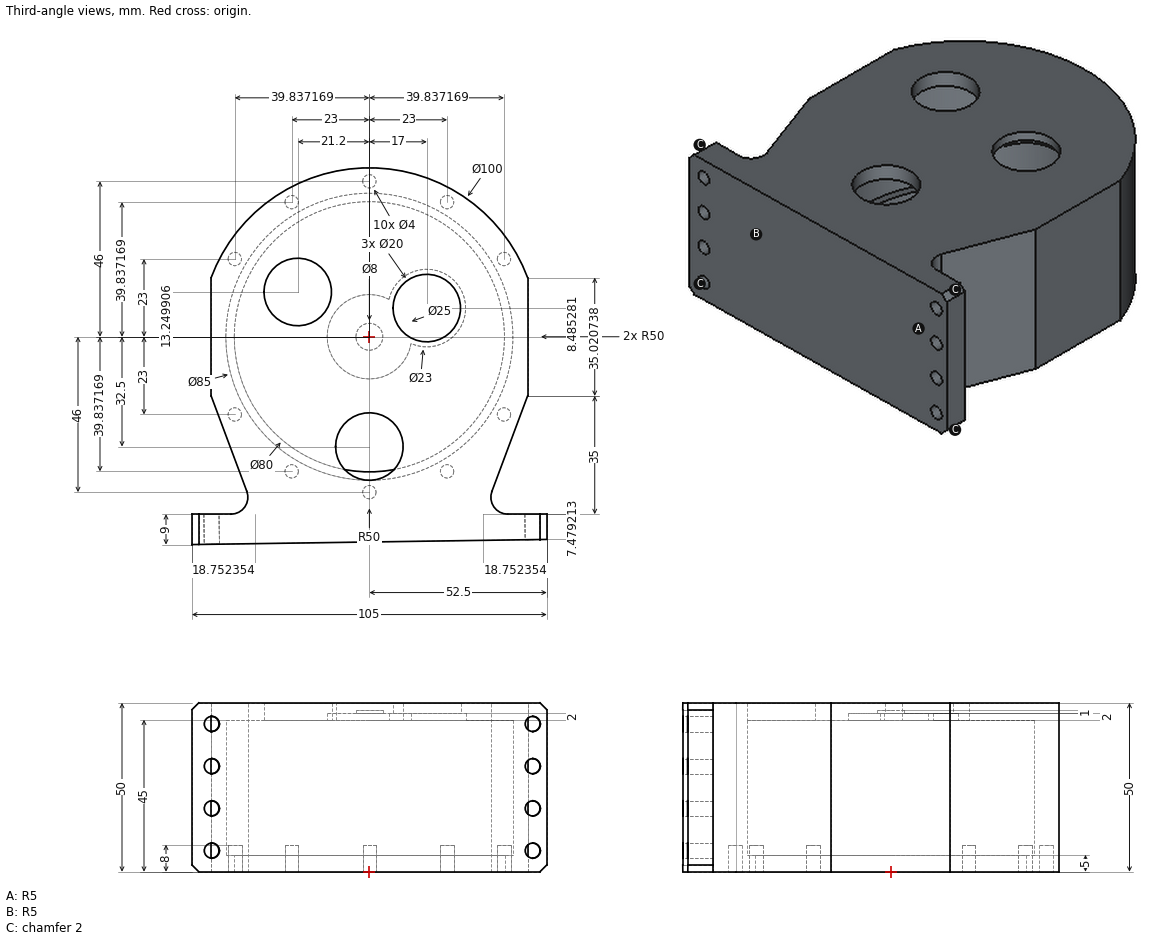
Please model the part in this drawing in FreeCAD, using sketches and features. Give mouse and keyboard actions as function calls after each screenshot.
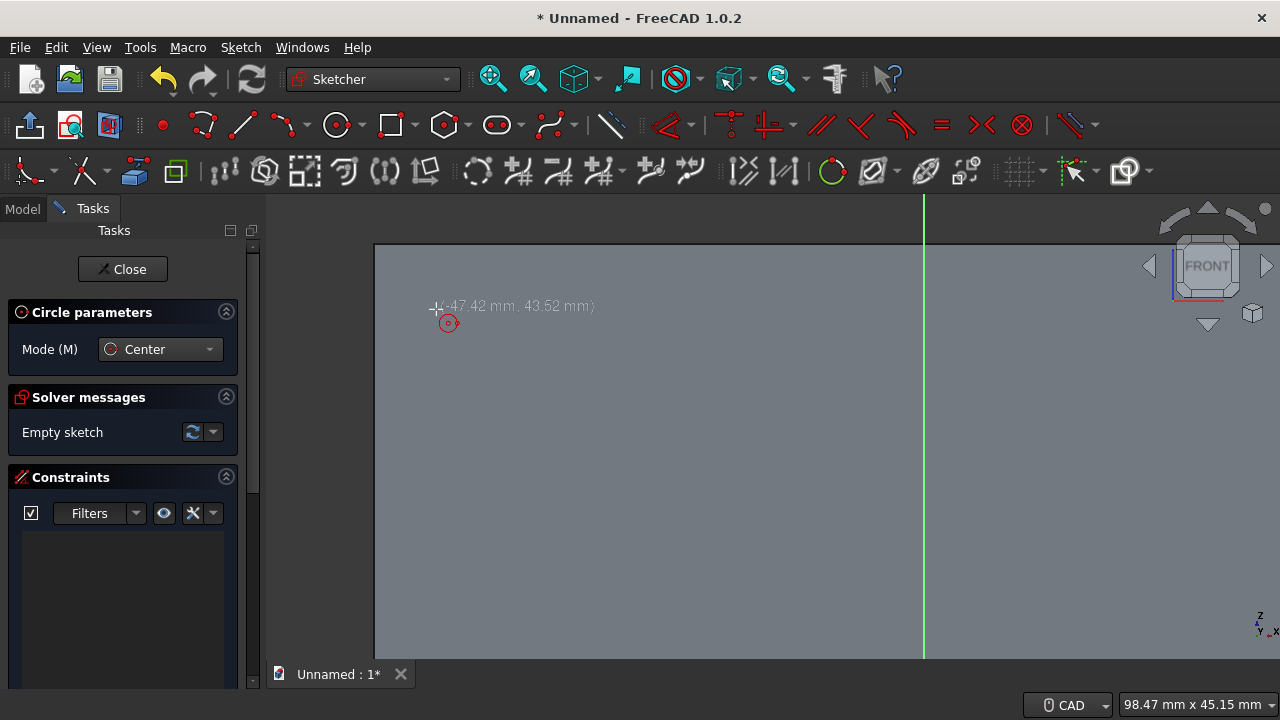
click(435, 308)
click(451, 292)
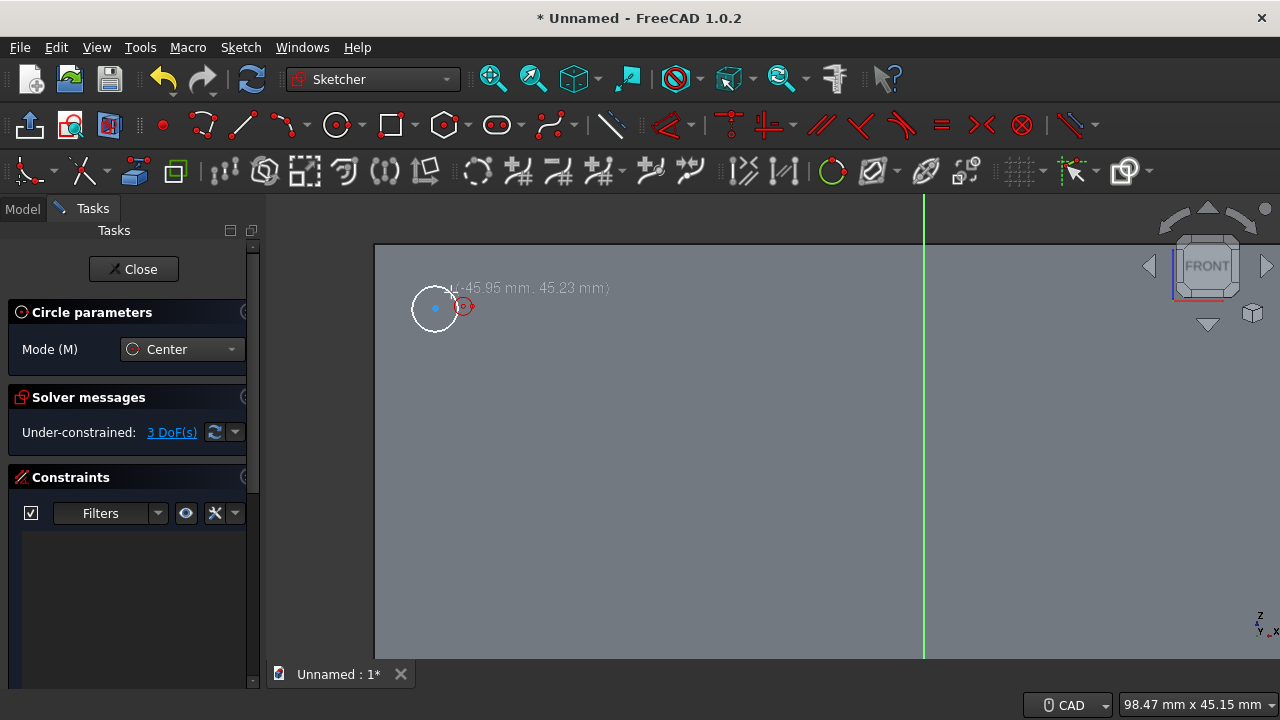
click(435, 437)
click(451, 421)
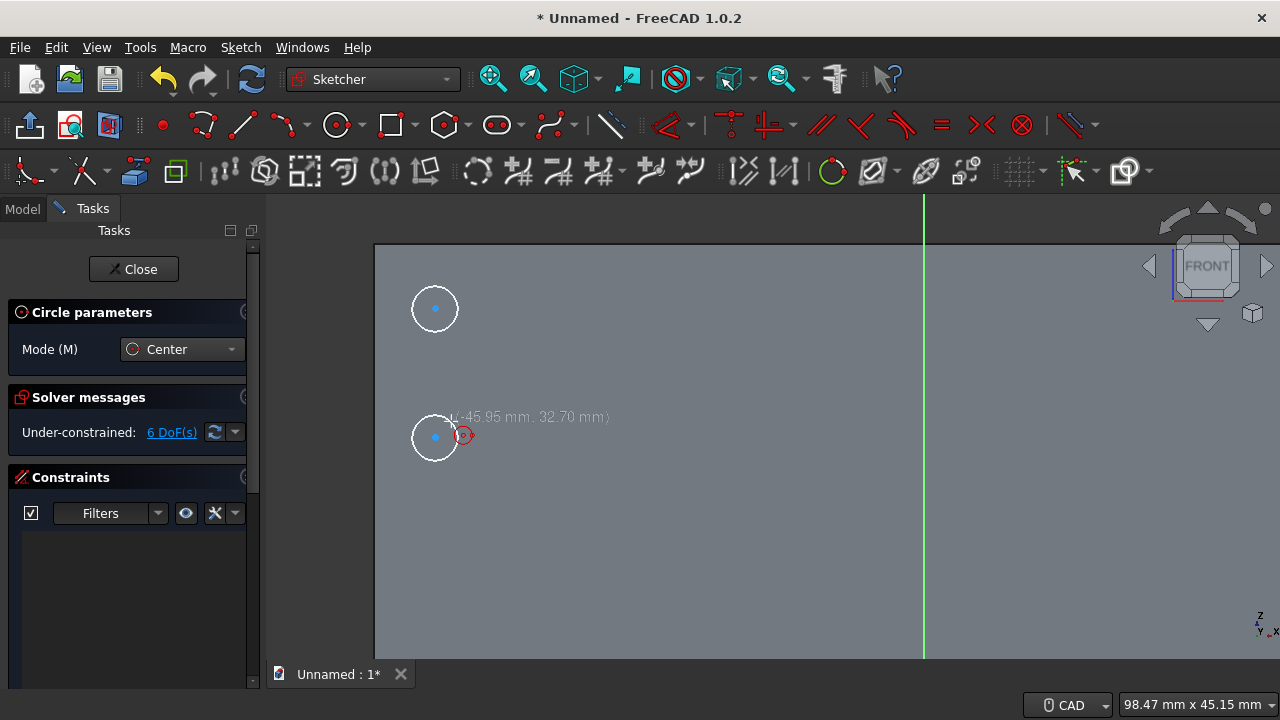
scroll(437, 310, down, 3)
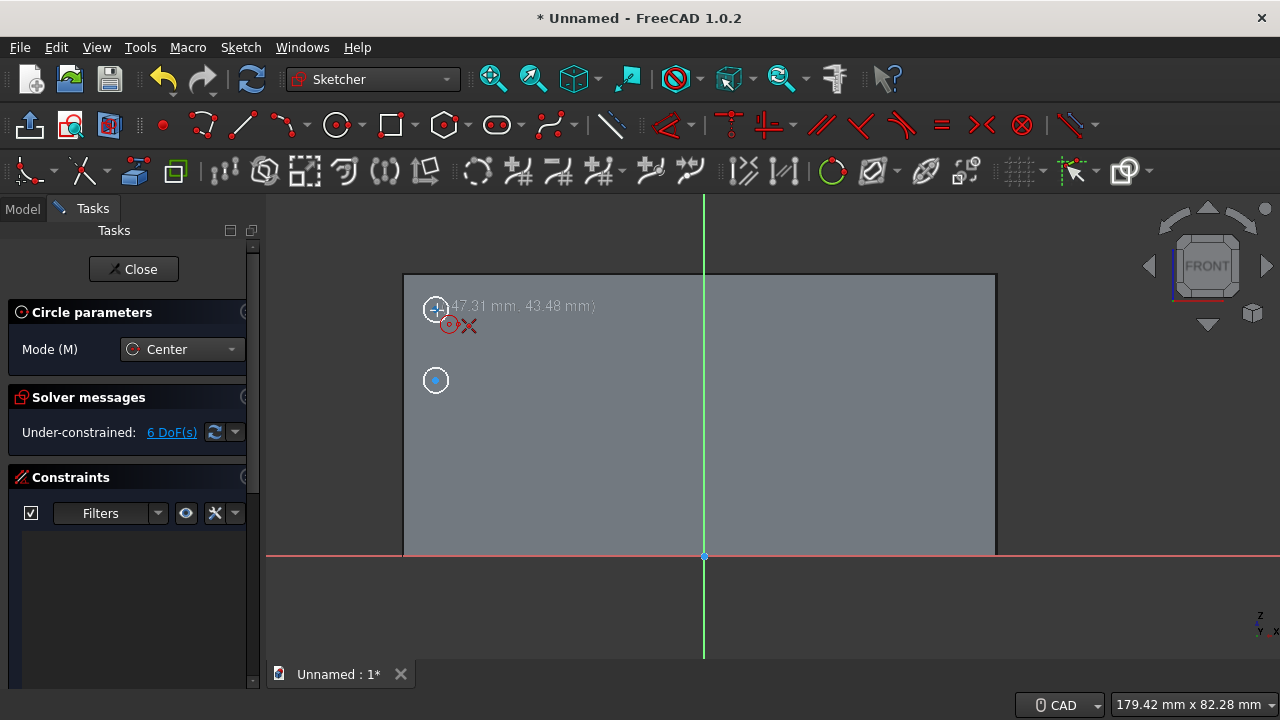
scroll(973, 380, up, 3)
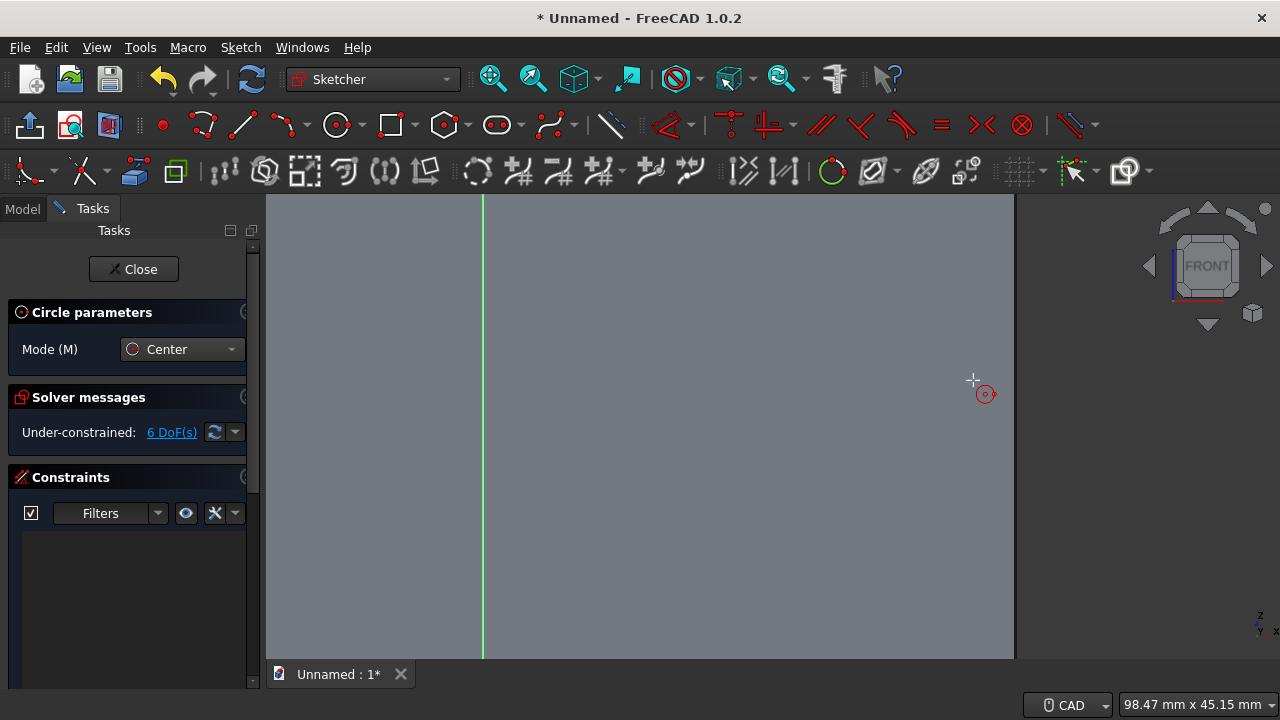
click(972, 379)
click(989, 363)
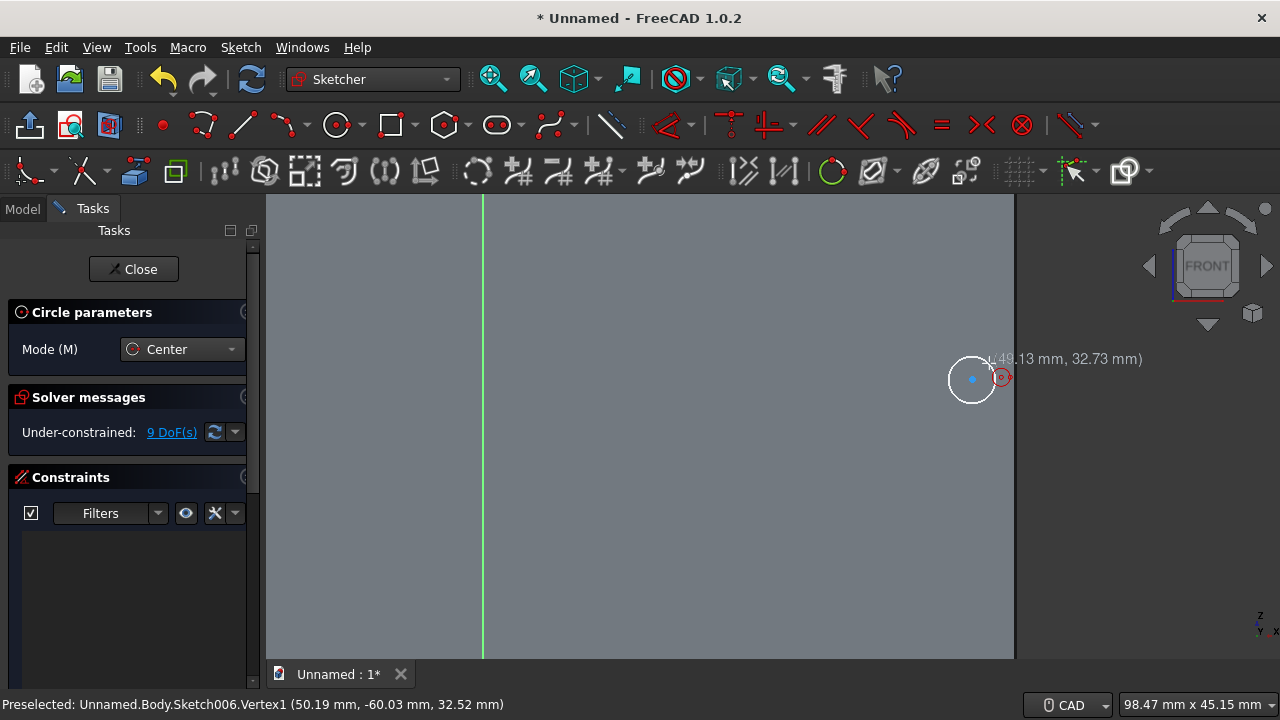
click(972, 251)
click(989, 234)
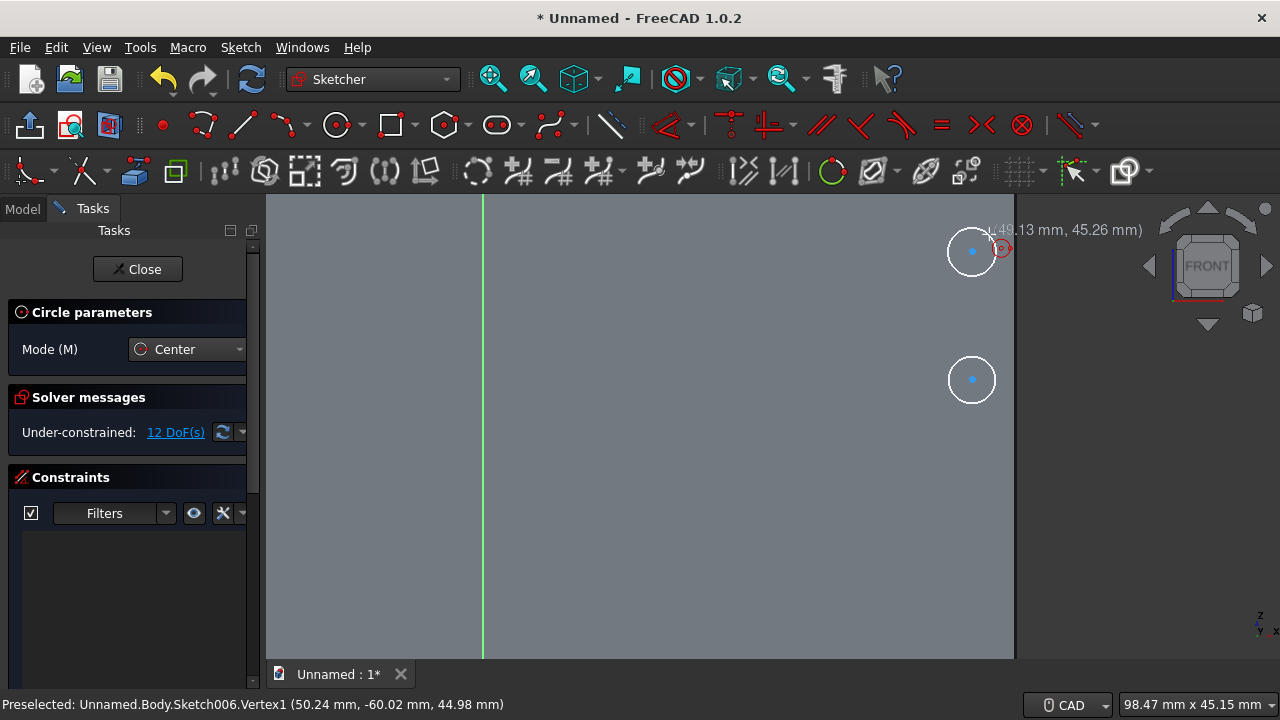
click(972, 508)
click(989, 492)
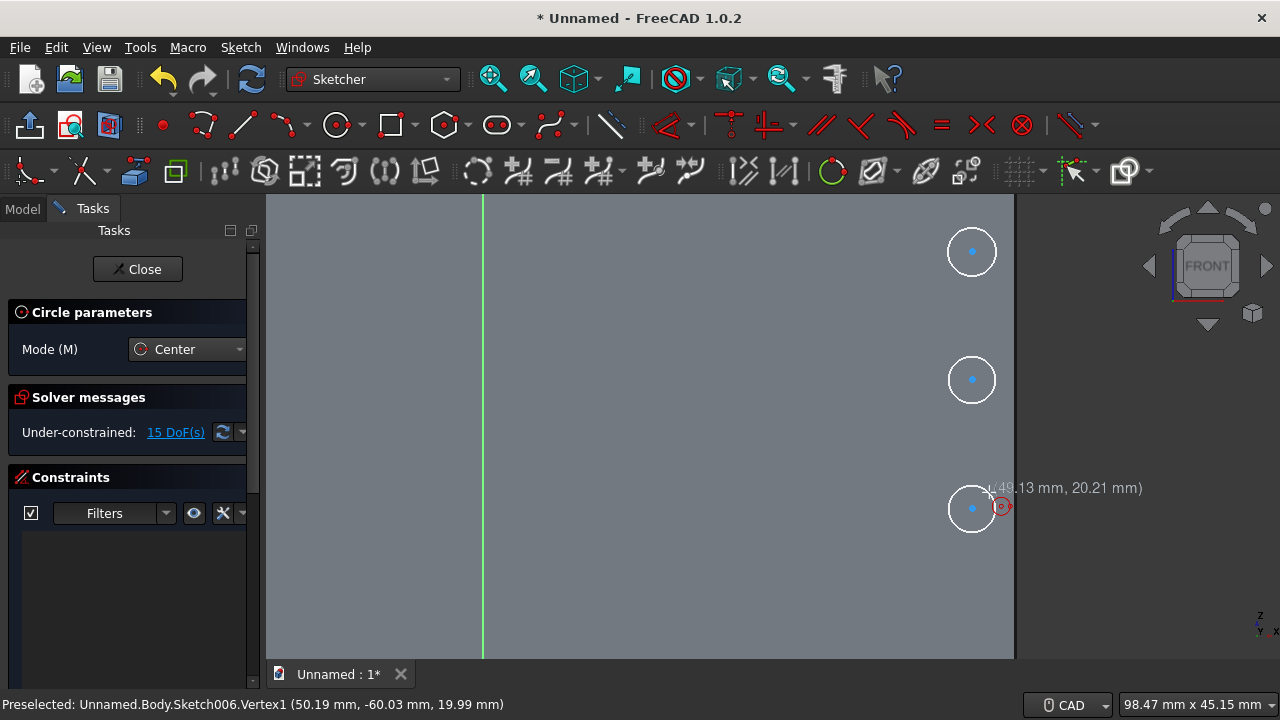
scroll(974, 381, down, 3)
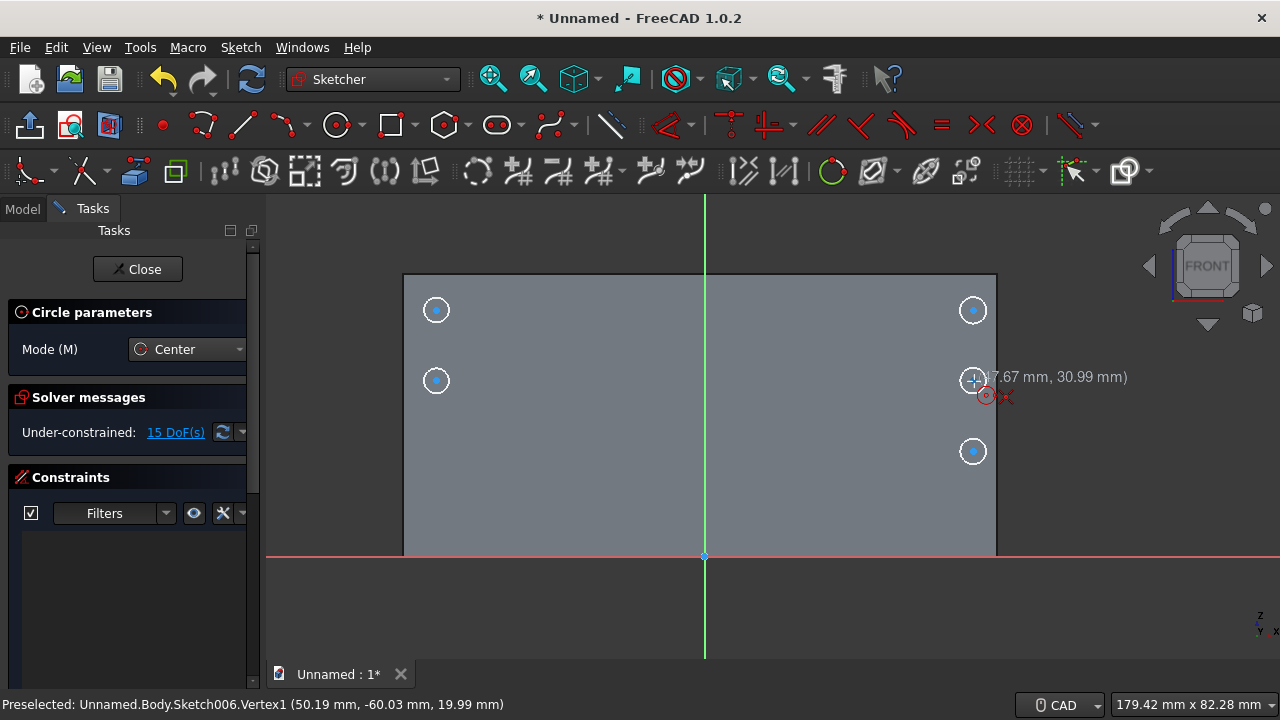
scroll(973, 522, up, 3)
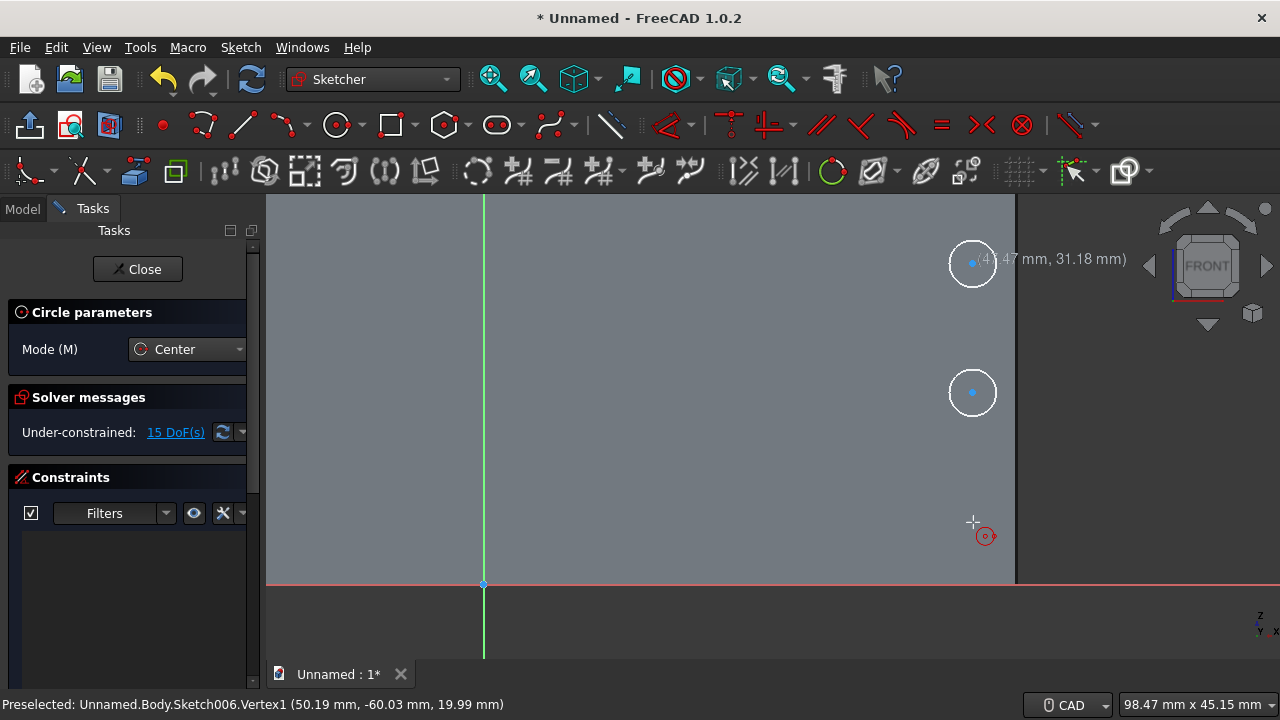
click(973, 521)
click(989, 504)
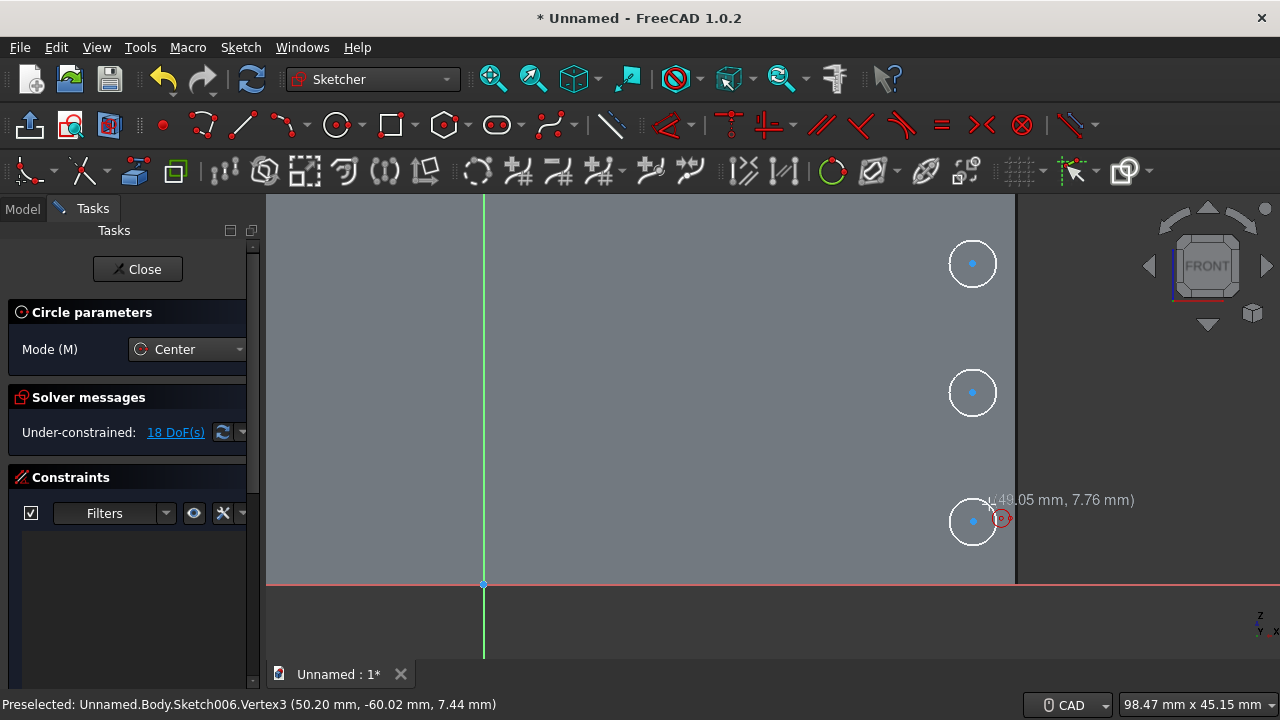
scroll(973, 522, down, 3)